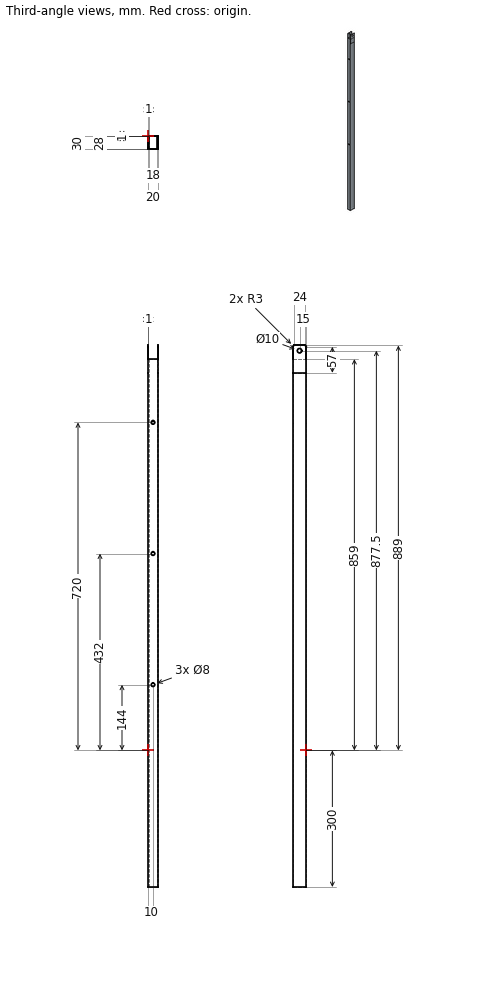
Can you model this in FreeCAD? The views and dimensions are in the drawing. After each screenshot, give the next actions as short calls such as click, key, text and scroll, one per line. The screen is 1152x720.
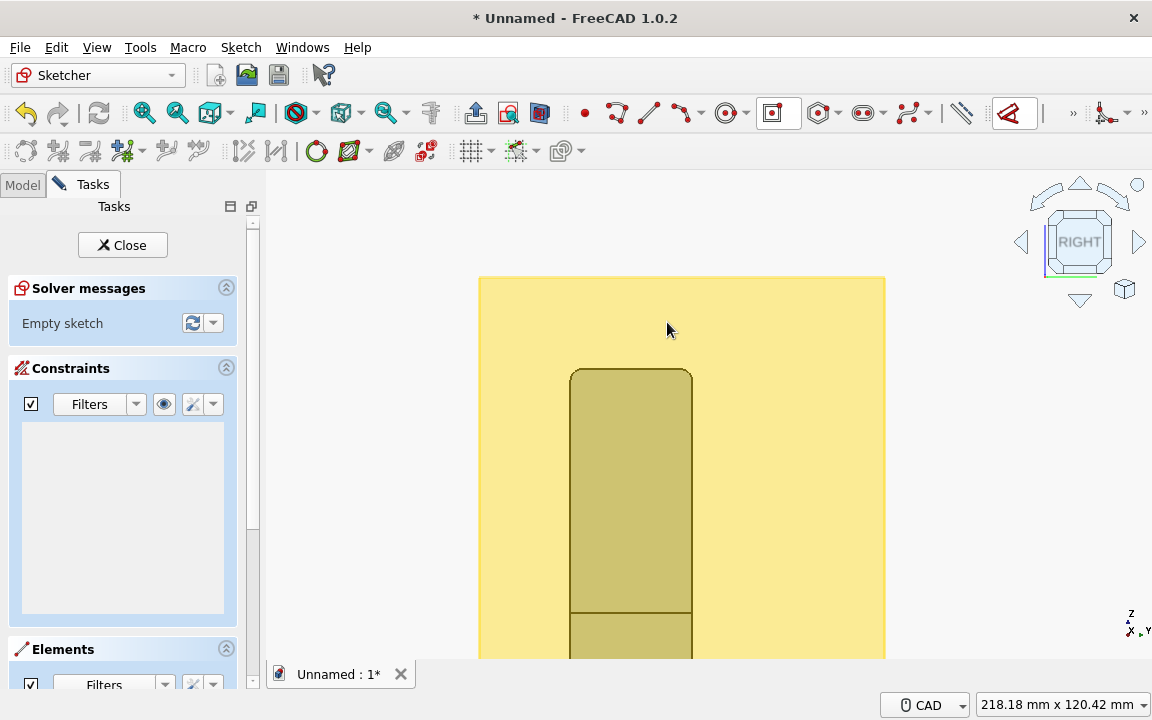
scroll(630, 416, up, 10)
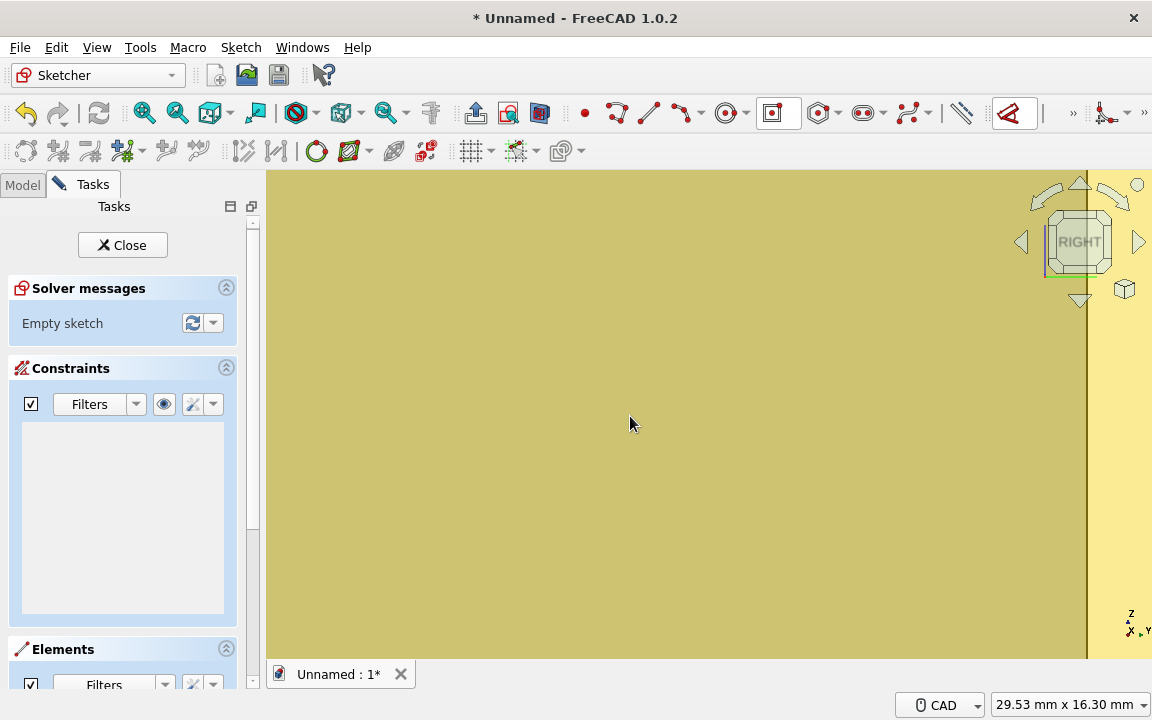
key(g)
key(c)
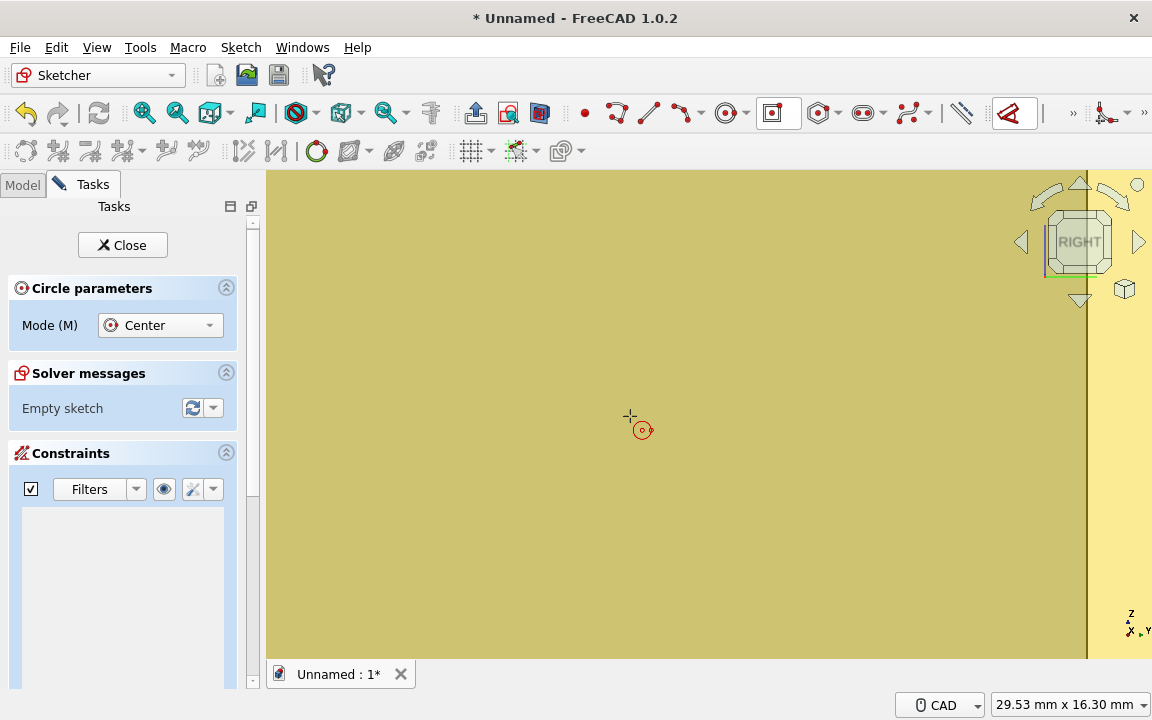
click(637, 410)
click(743, 304)
key(Escape)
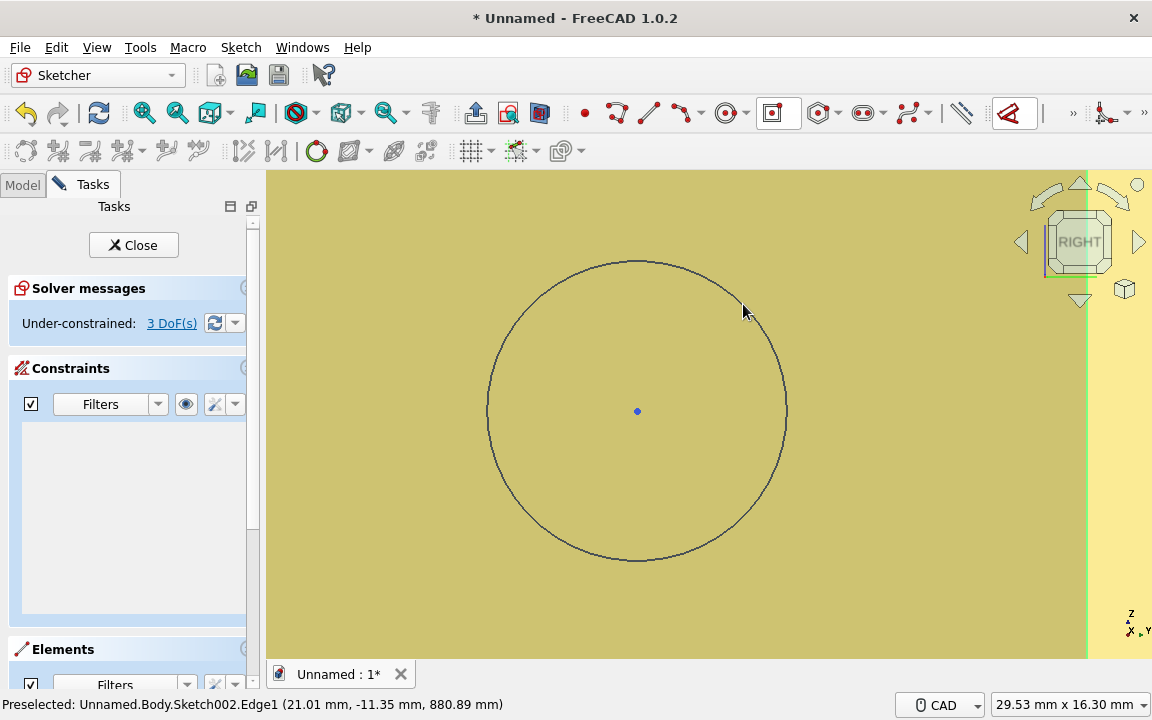
click(743, 305)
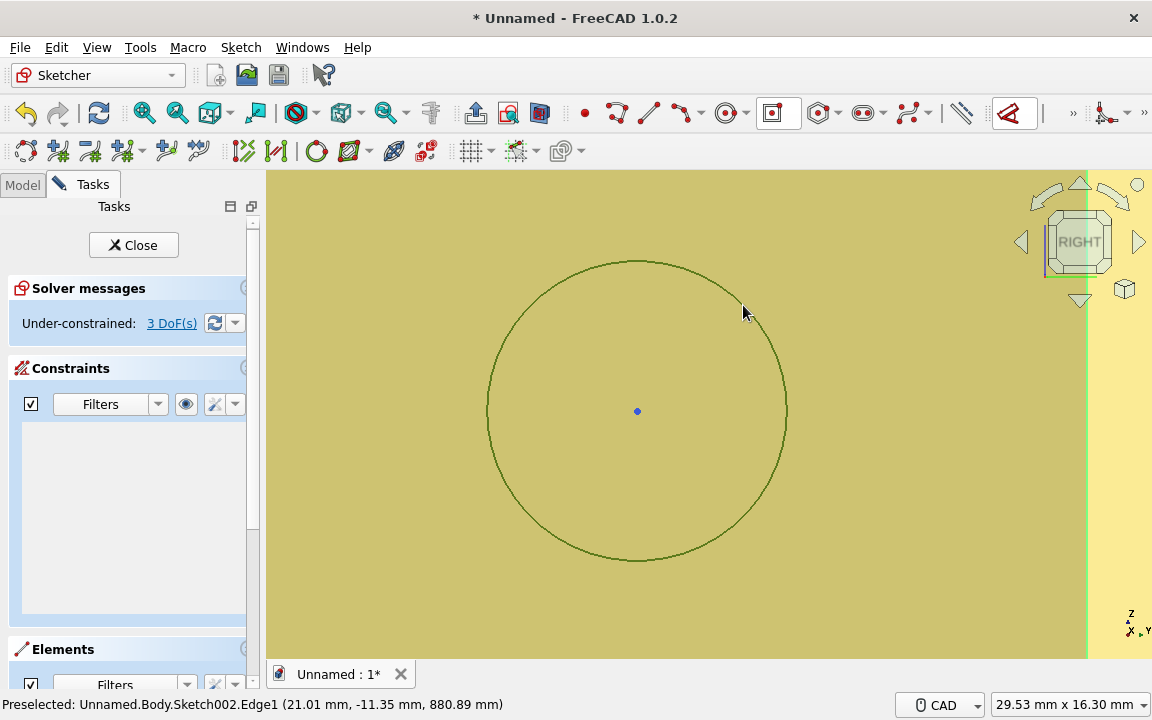
click(1032, 114)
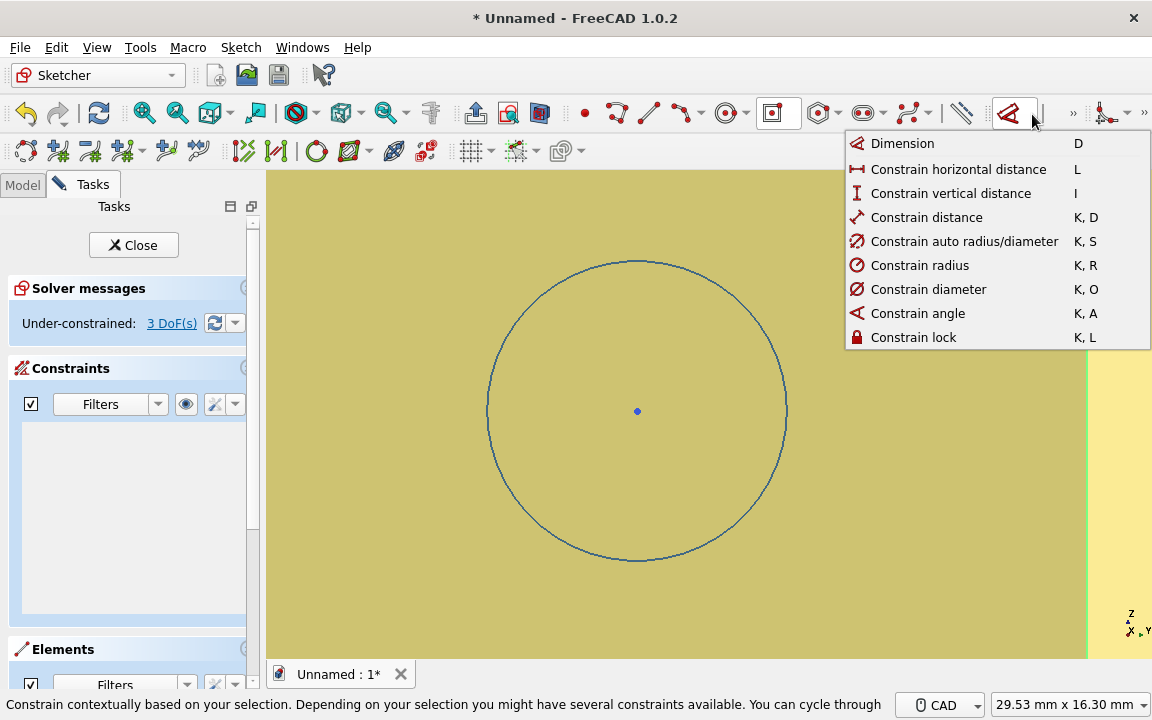
click(998, 289)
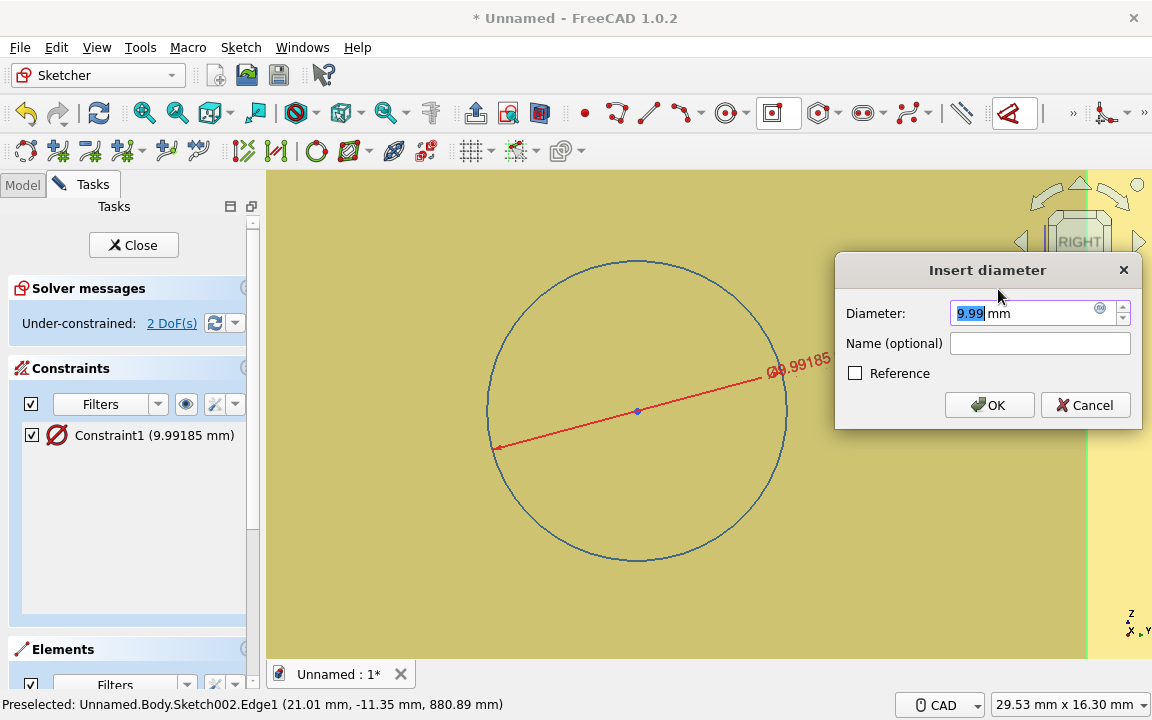
text(10)
key(Return)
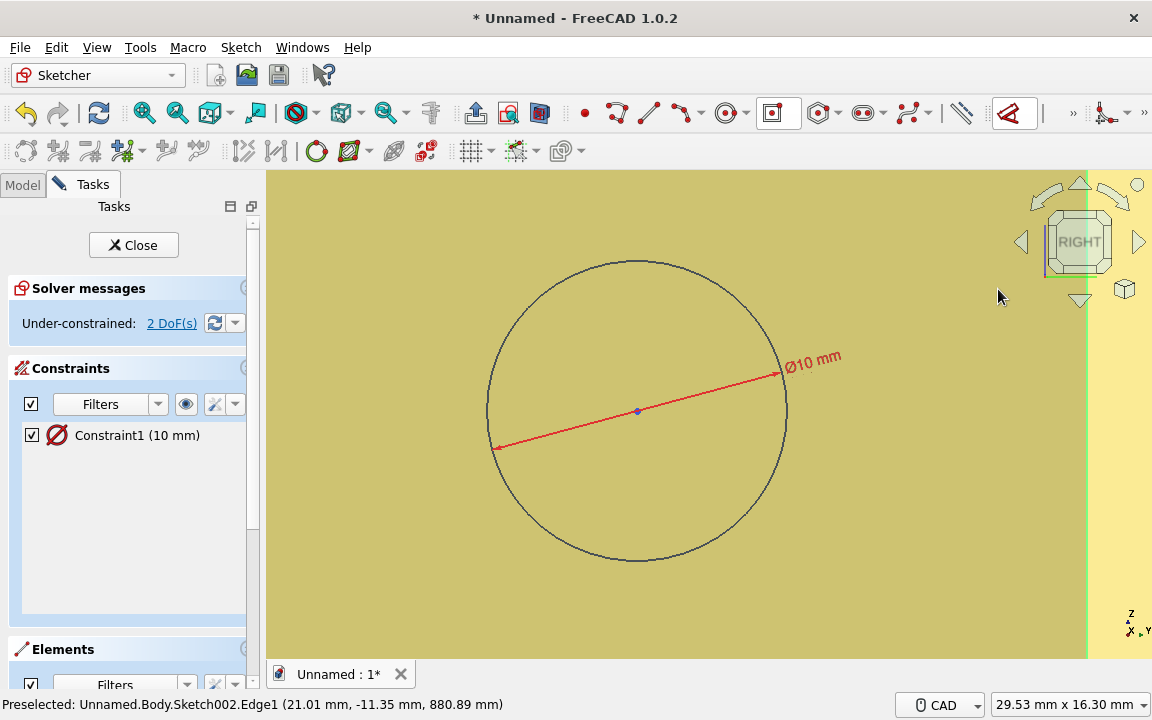
click(637, 411)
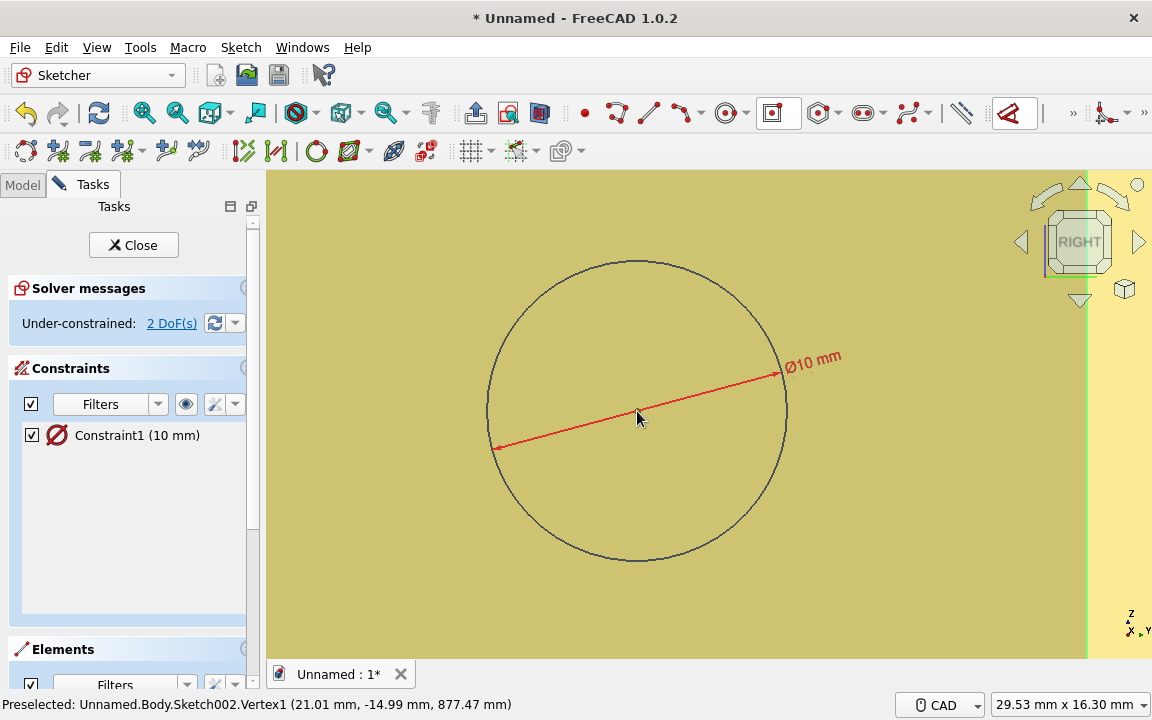
click(1032, 114)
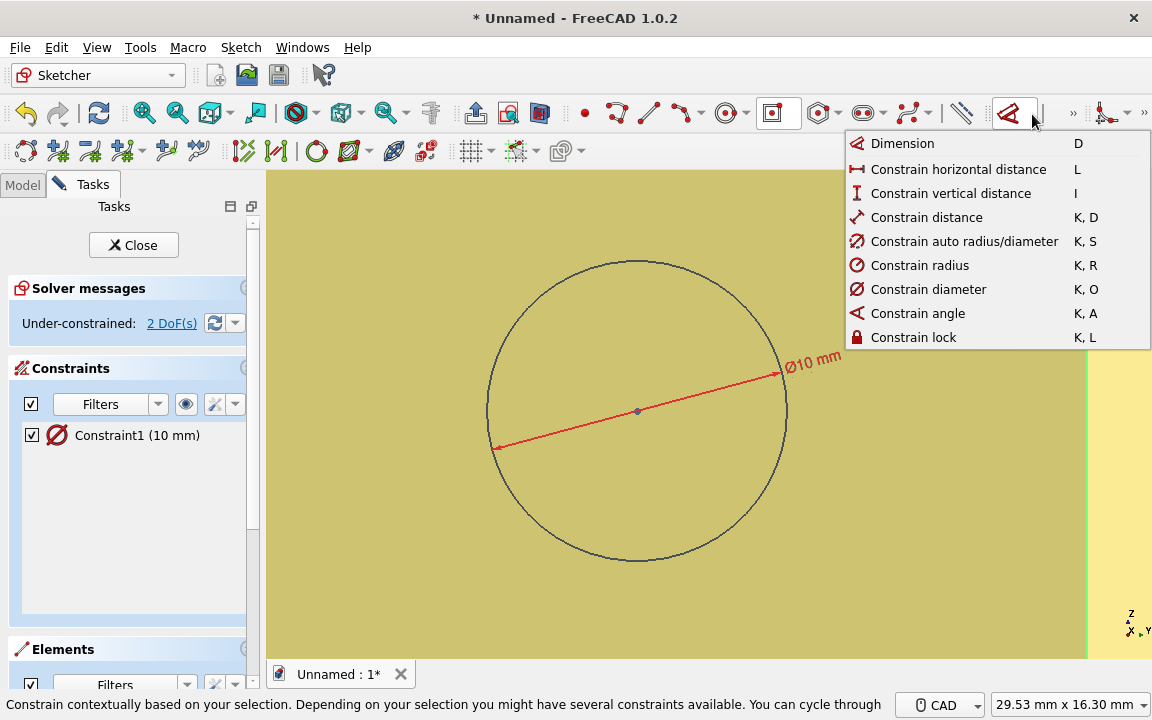
click(998, 169)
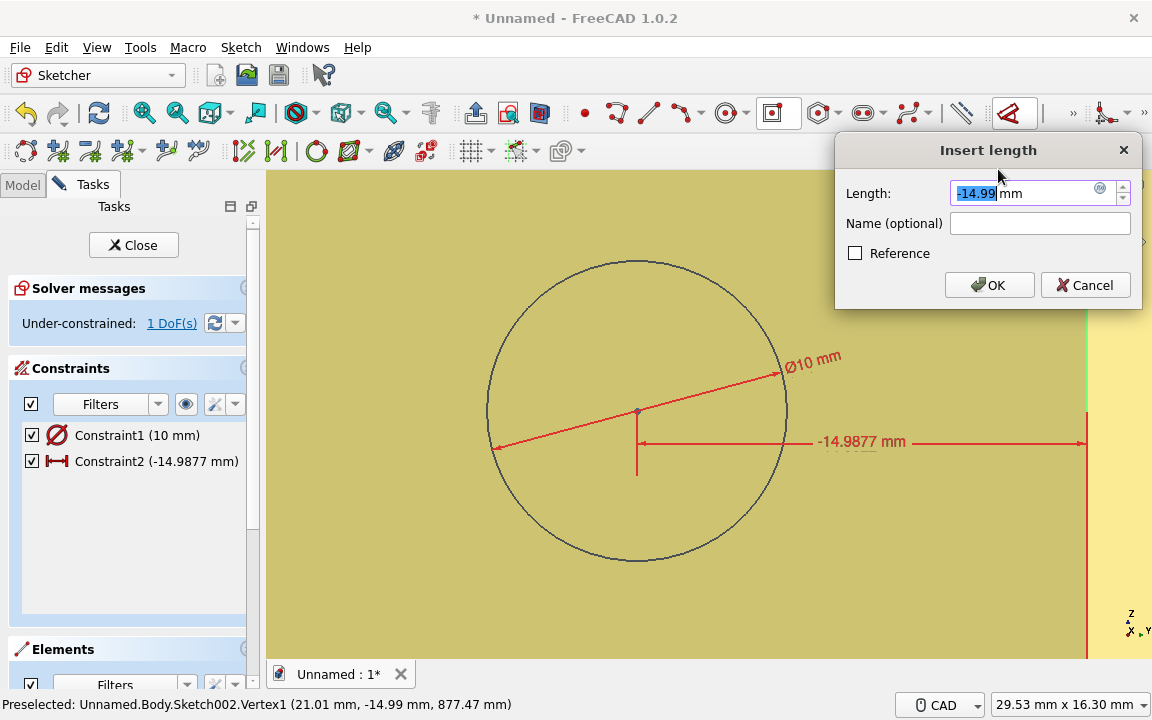
text(-15)
key(Return)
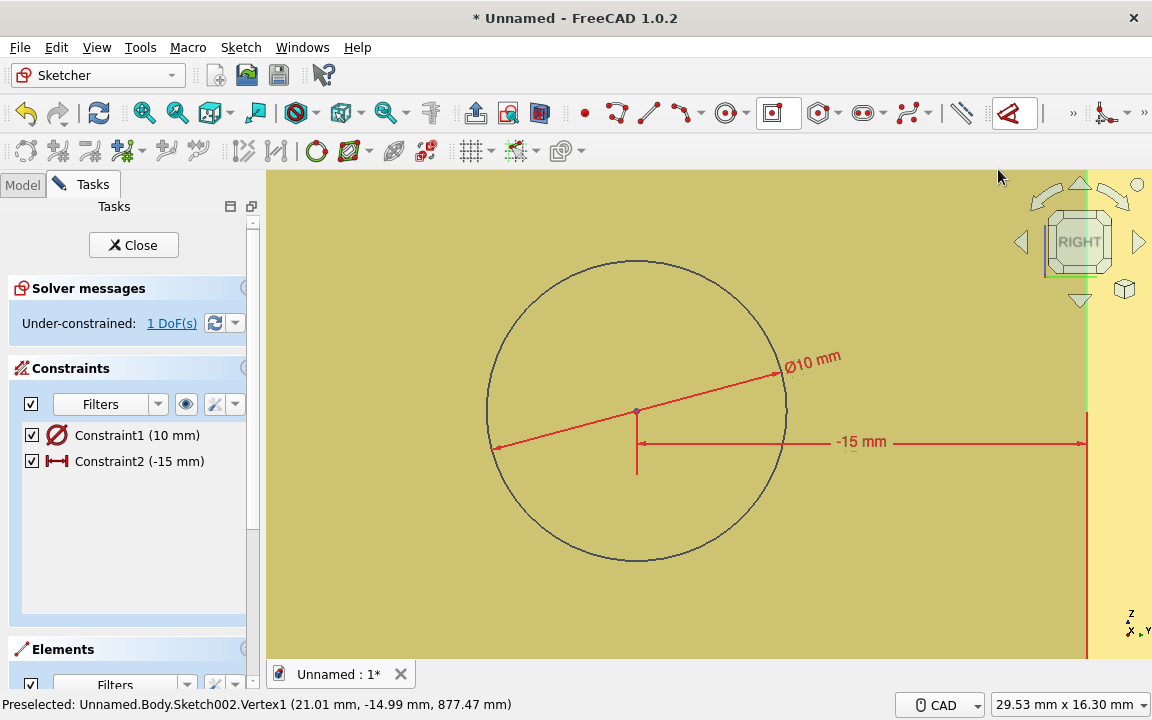
click(637, 411)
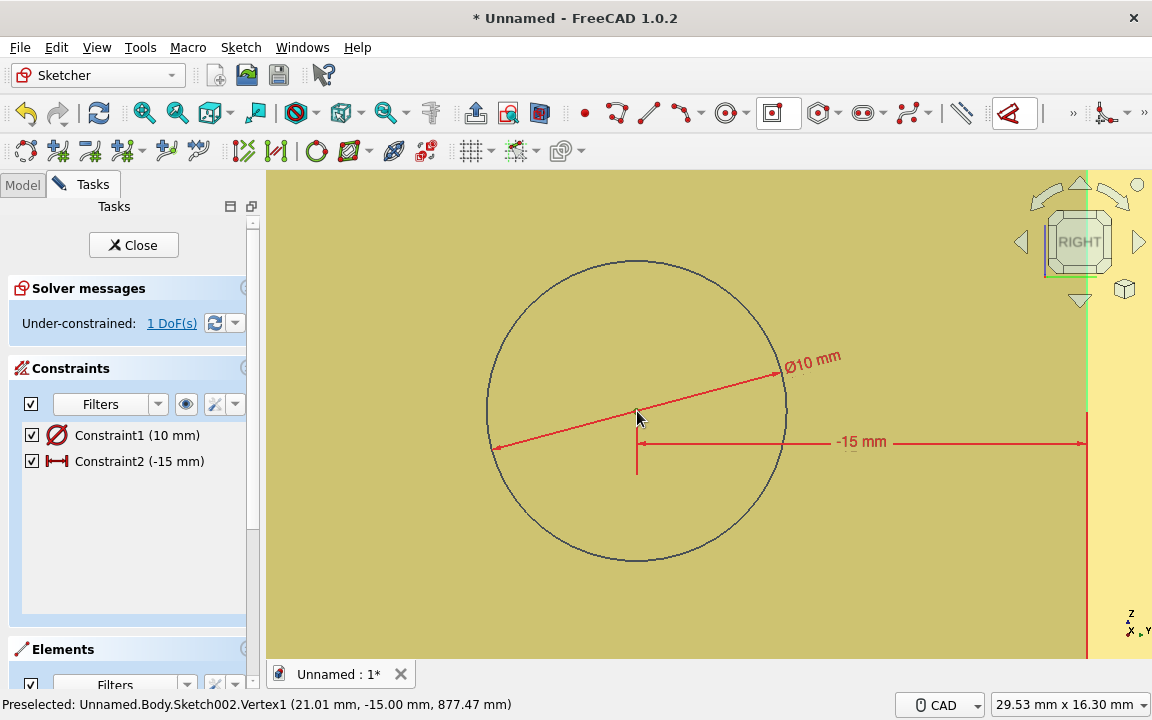
key(i)